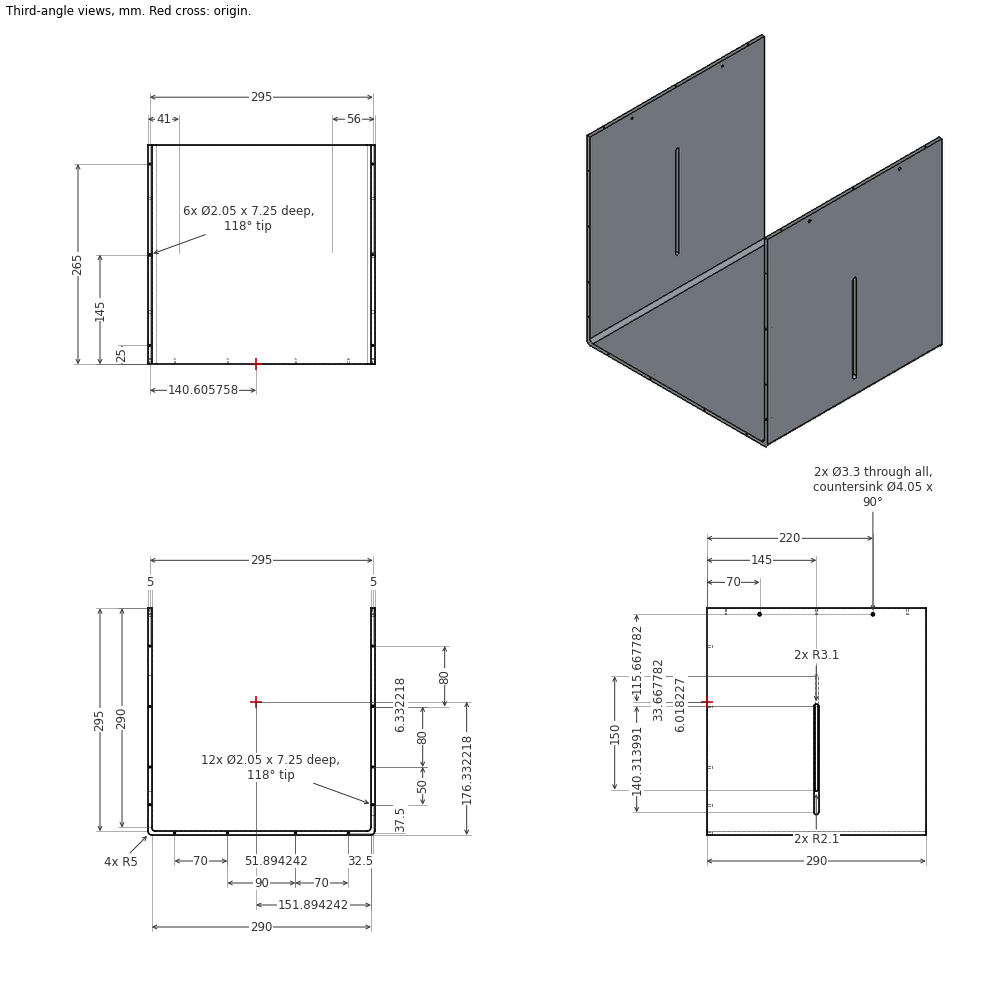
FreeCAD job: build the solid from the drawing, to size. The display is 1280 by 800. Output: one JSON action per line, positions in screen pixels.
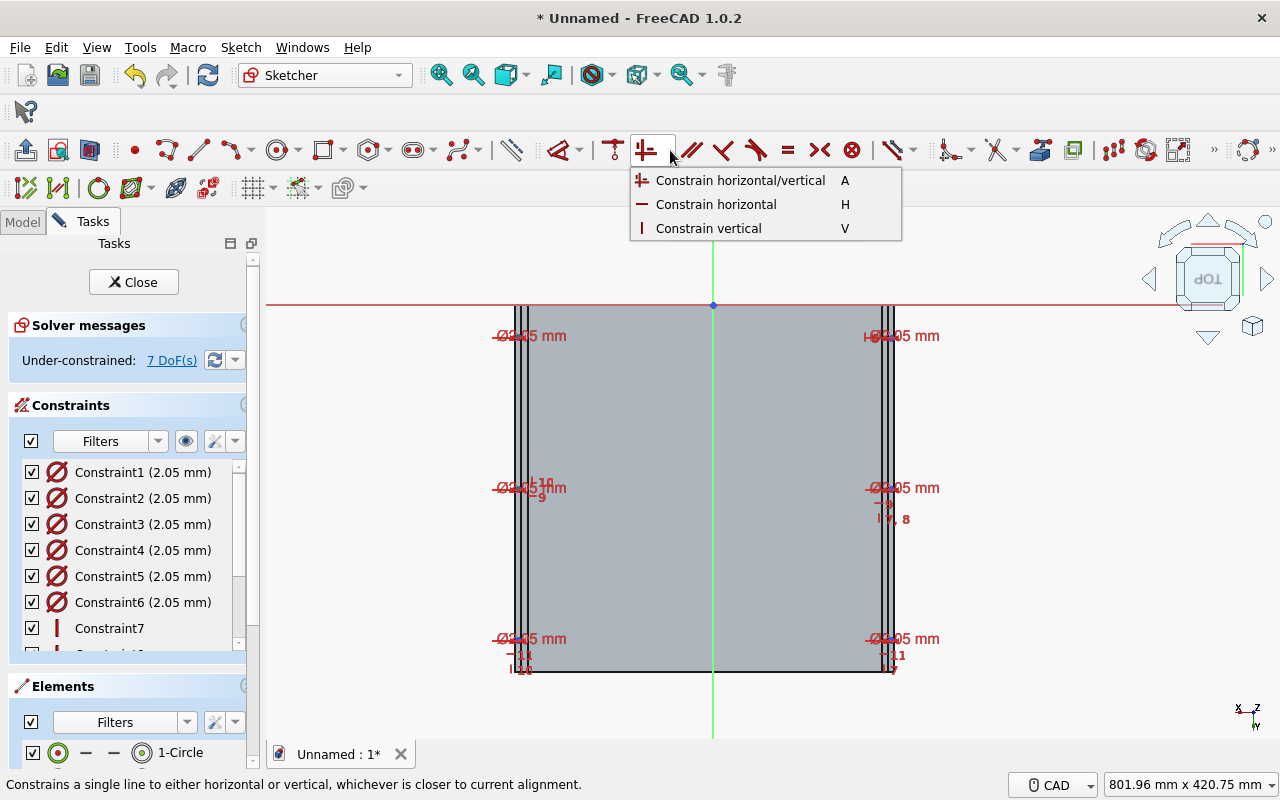
{"action": "left_click", "coordinate": [766, 228]}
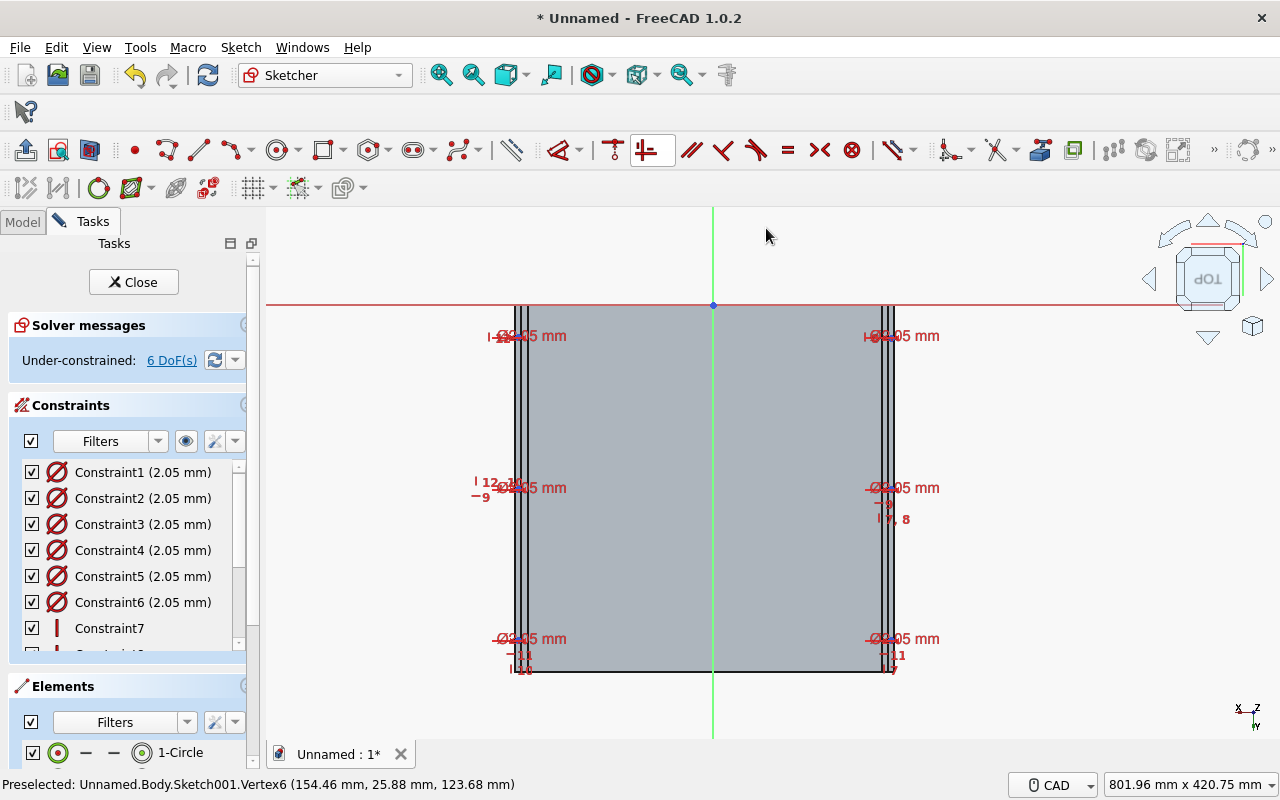
{"action": "left_click", "coordinate": [891, 338]}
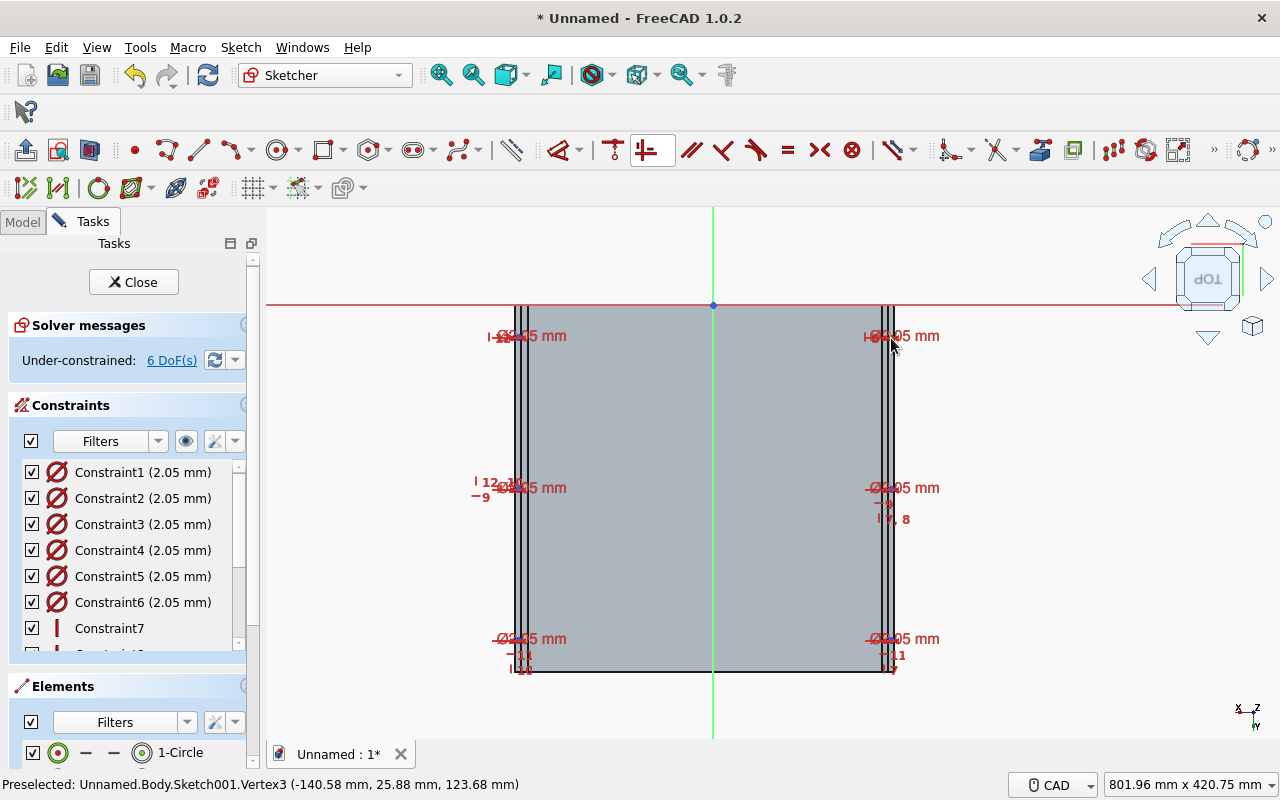
{"action": "left_click", "coordinate": [518, 338]}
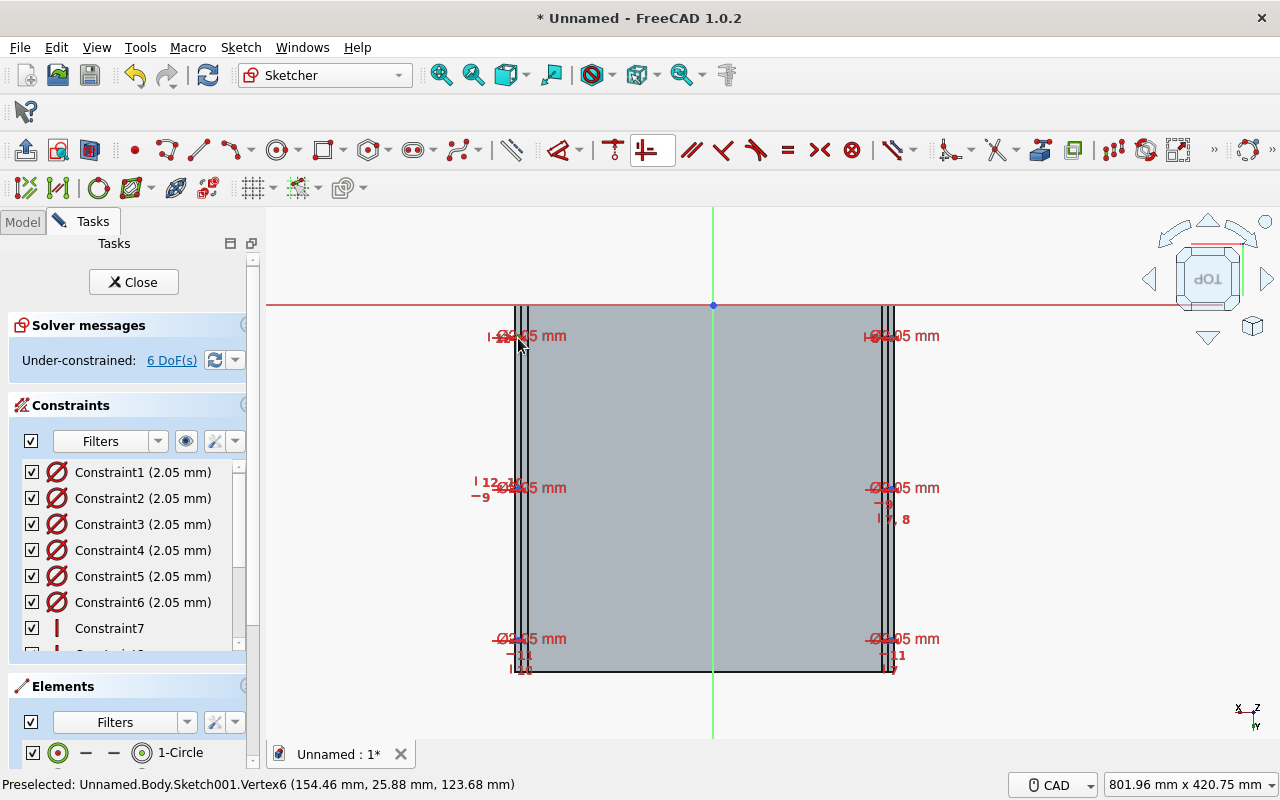
{"action": "left_click", "coordinate": [670, 150]}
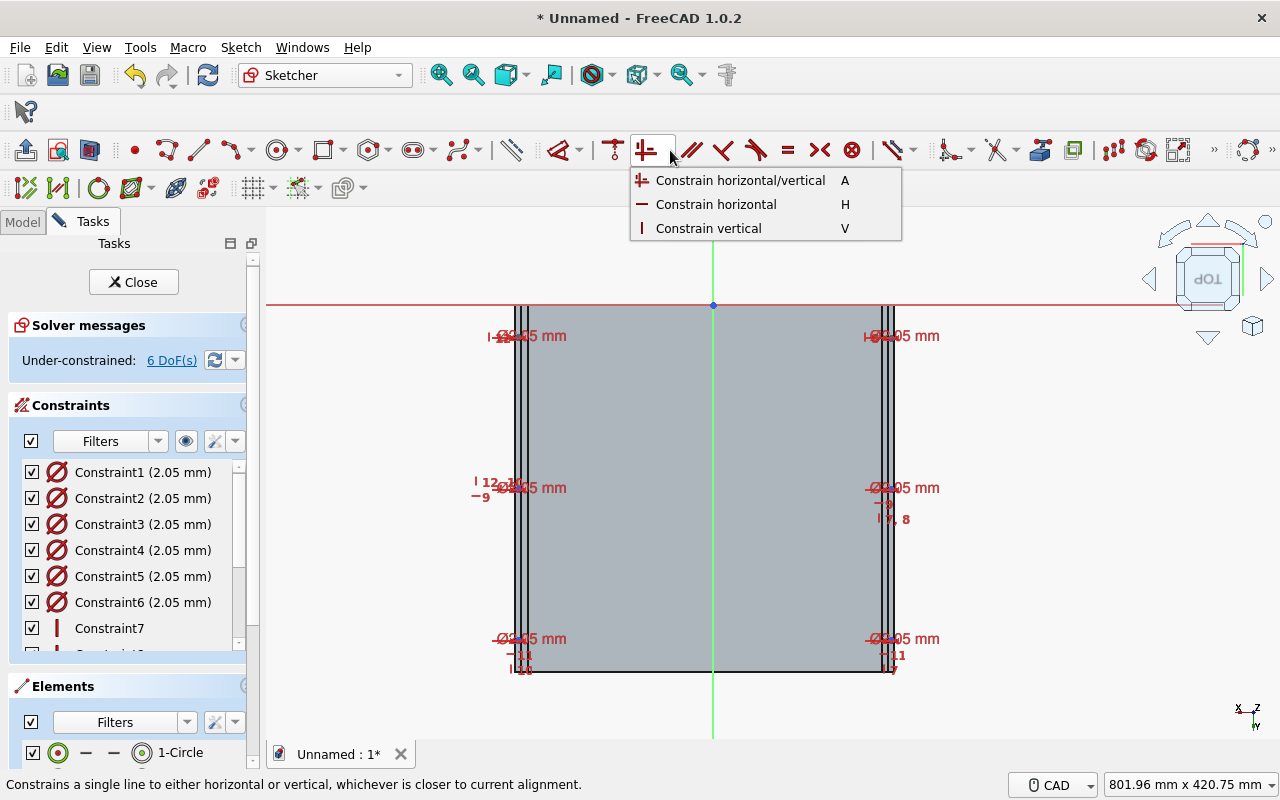
{"action": "left_click", "coordinate": [766, 204]}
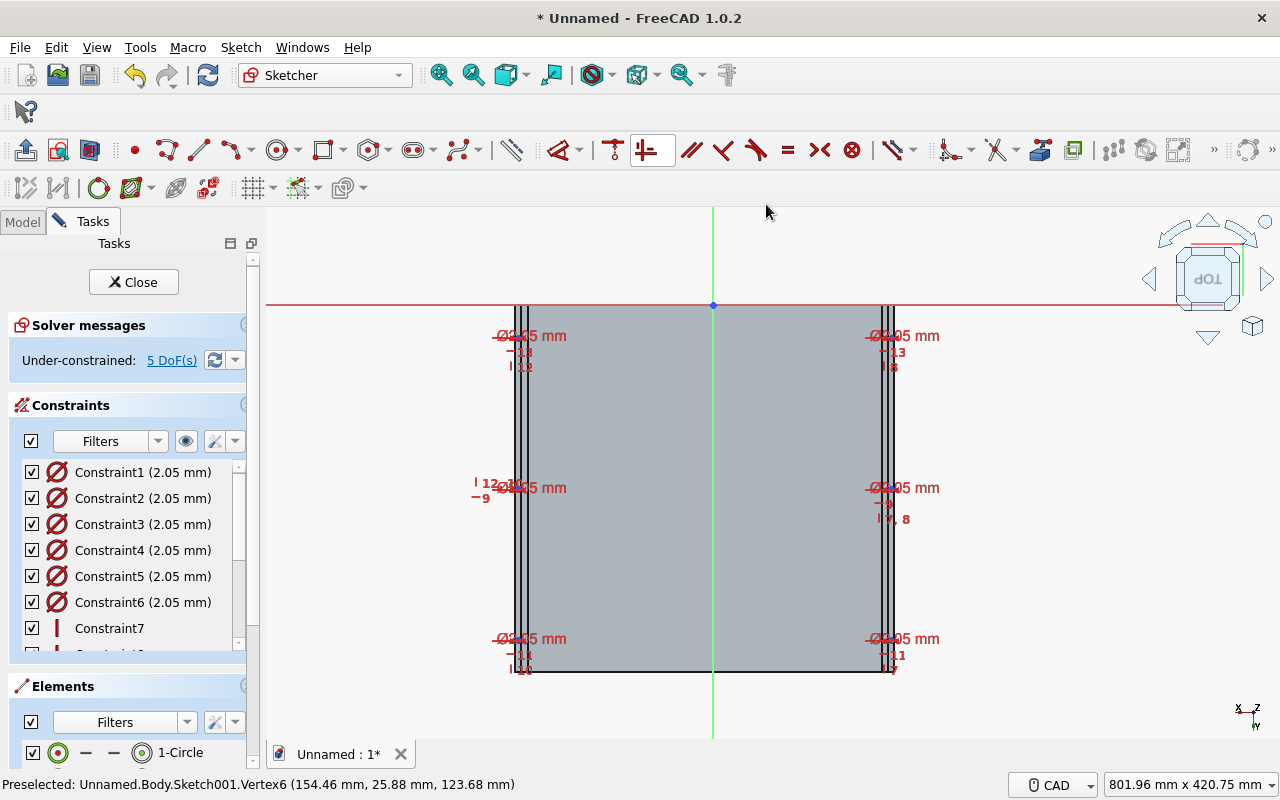
{"action": "left_click", "coordinate": [558, 150]}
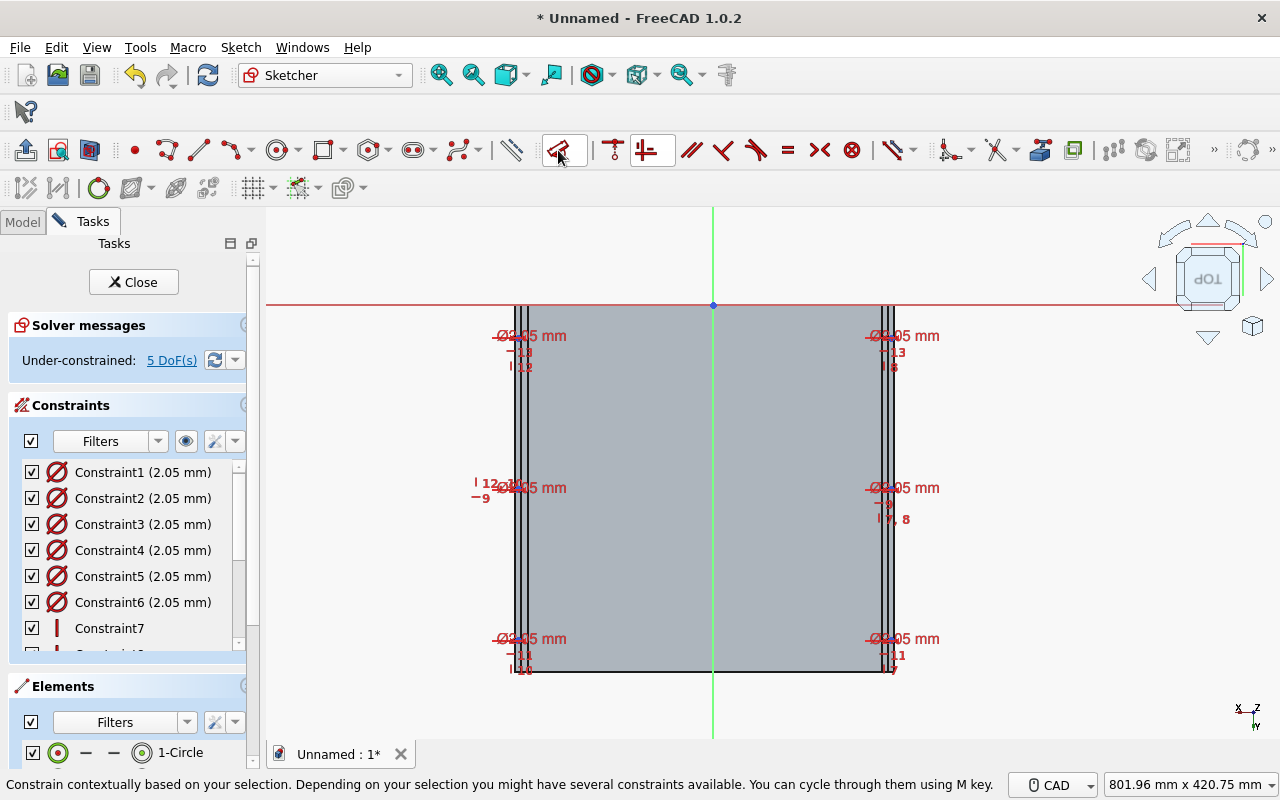
{"action": "scroll", "coordinate": [891, 338], "scroll_direction": "up", "scroll_amount": 2}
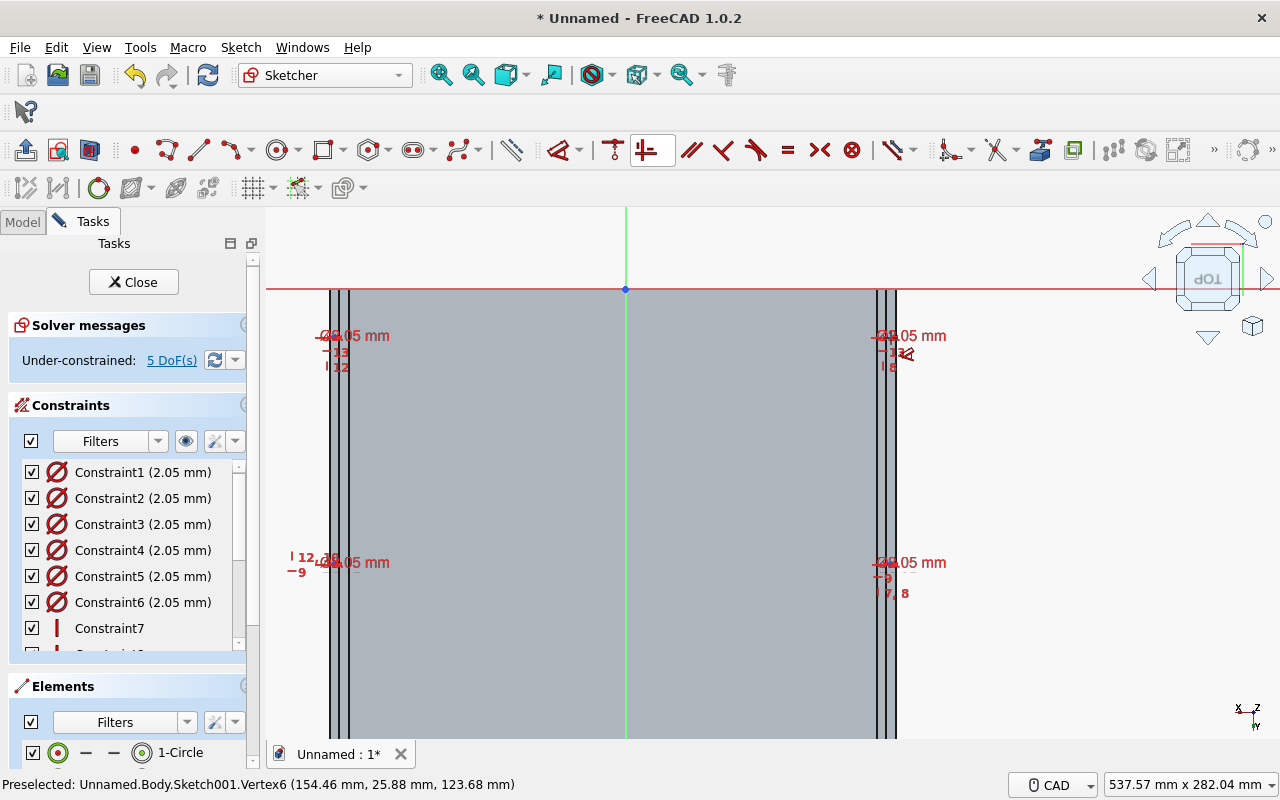
{"action": "left_click", "coordinate": [891, 338]}
{"action": "left_click", "coordinate": [925, 313]}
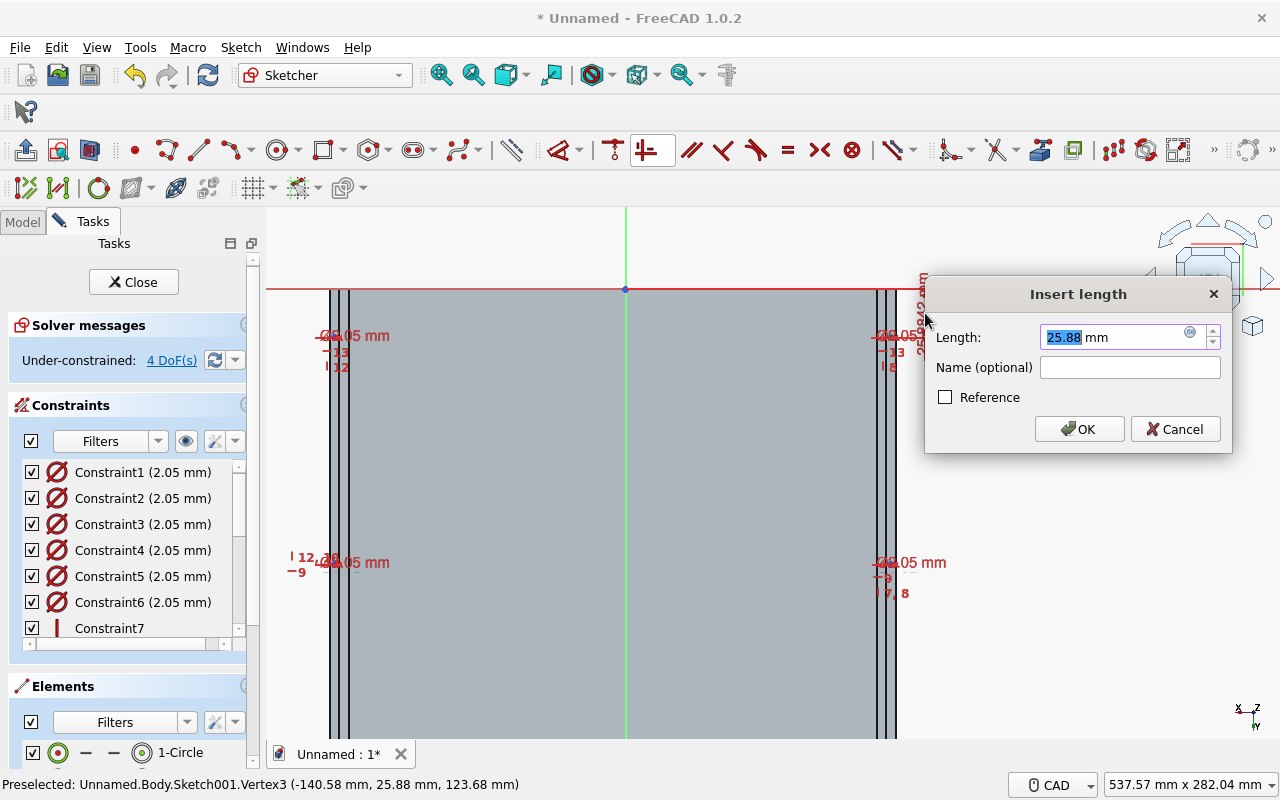
{"action": "type", "text": "25"}
{"action": "key", "text": "Return"}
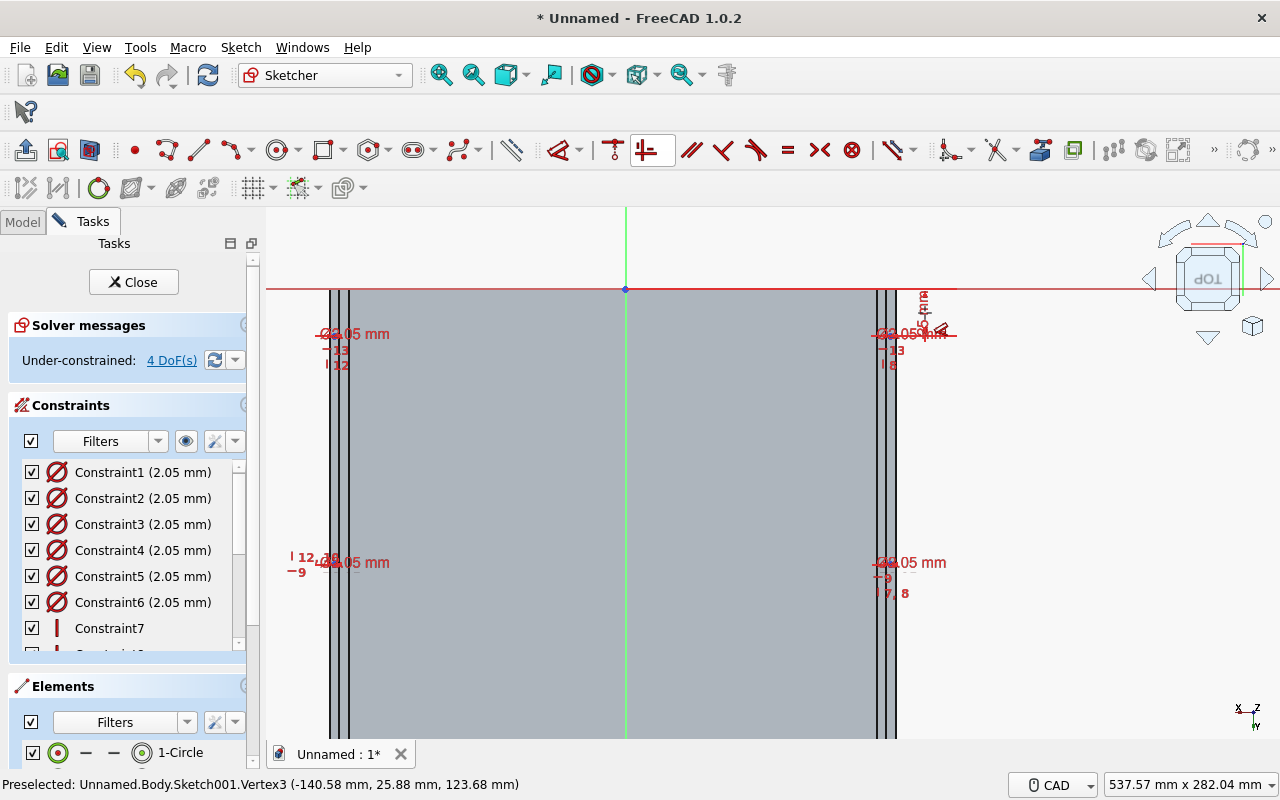
{"action": "left_click", "coordinate": [891, 565]}
{"action": "left_click", "coordinate": [925, 427]}